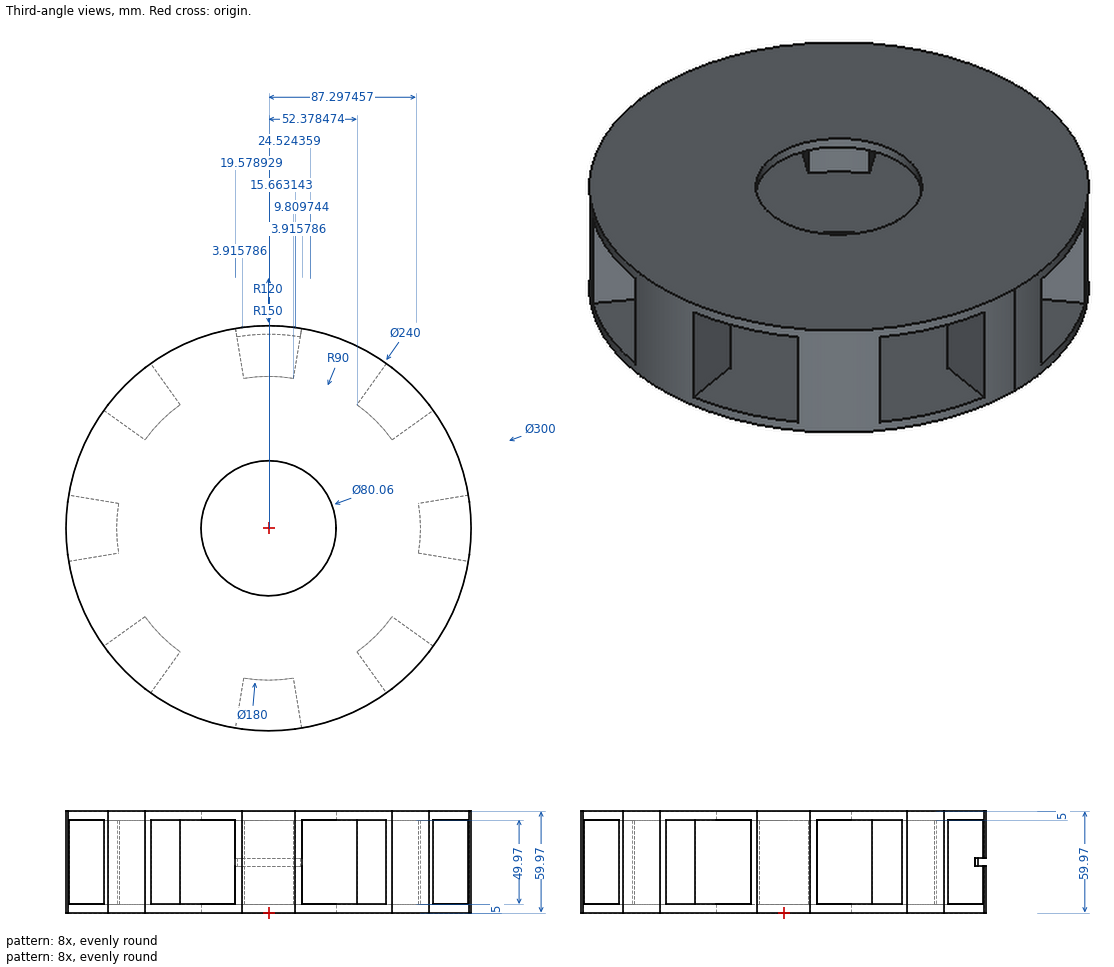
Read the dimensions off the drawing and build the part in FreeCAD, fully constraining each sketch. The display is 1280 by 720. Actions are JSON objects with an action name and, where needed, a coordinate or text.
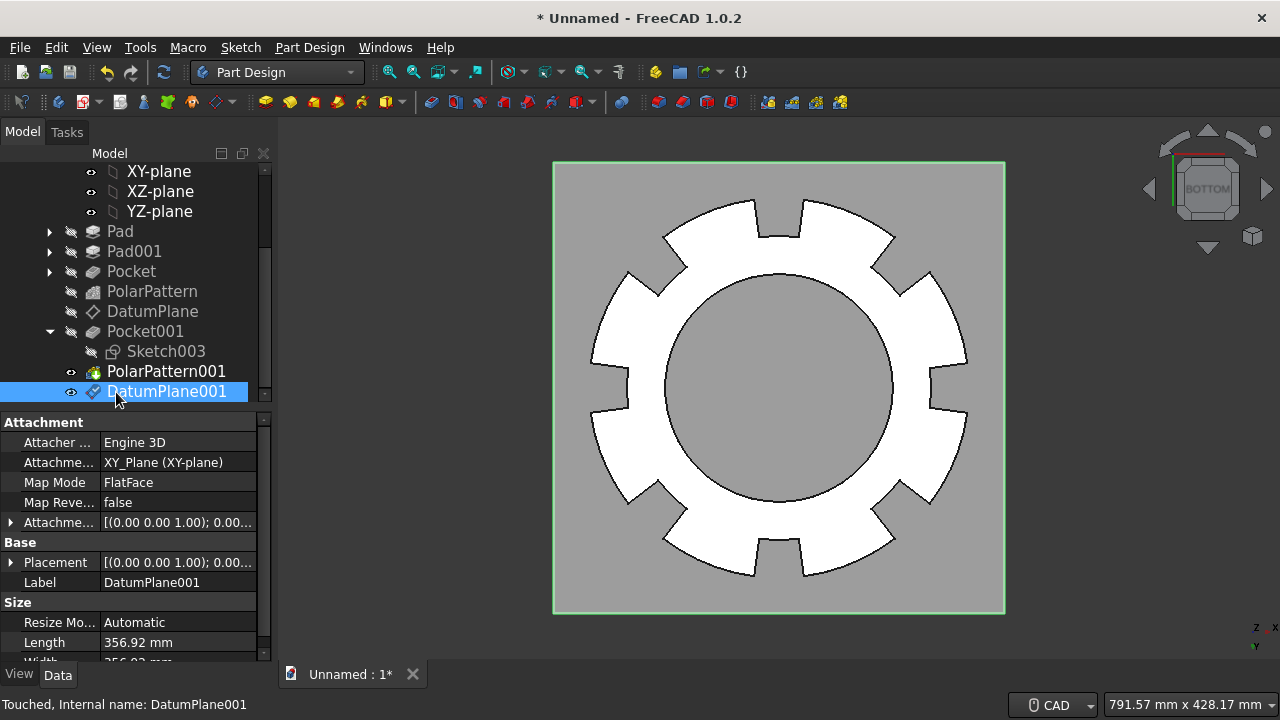
{"action": "left_click", "coordinate": [84, 102]}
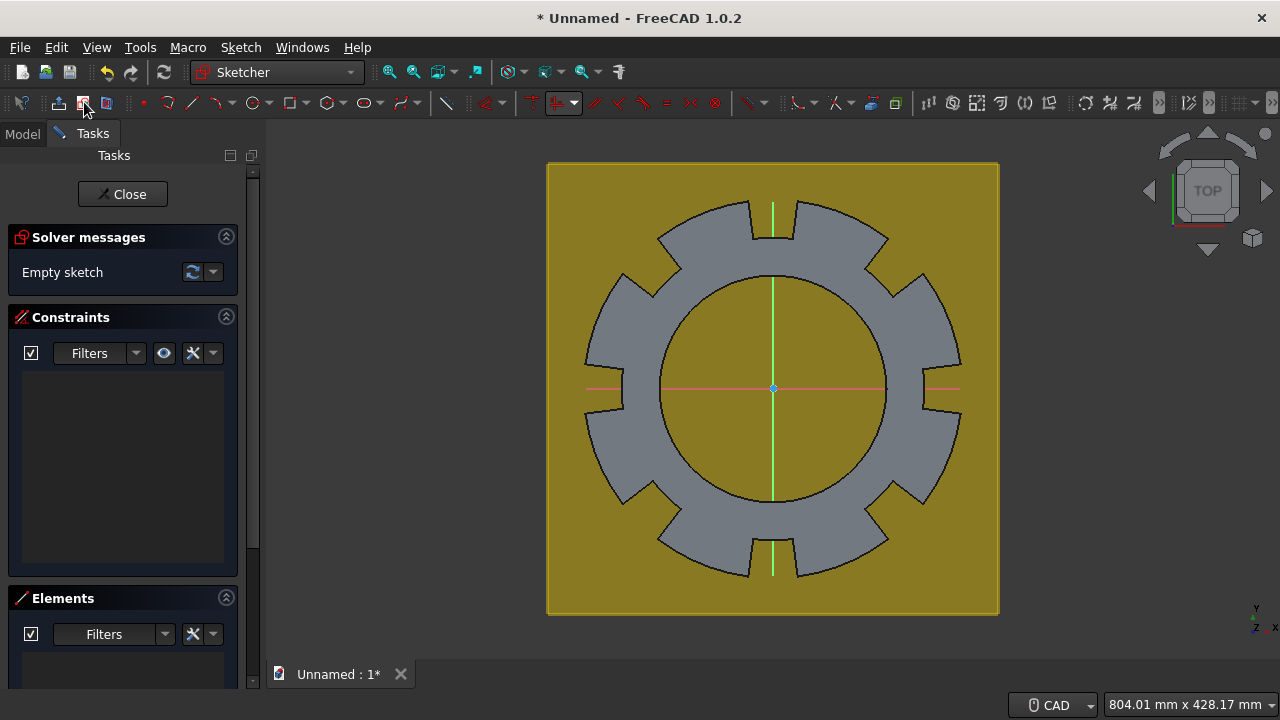
{"action": "left_click", "coordinate": [108, 104]}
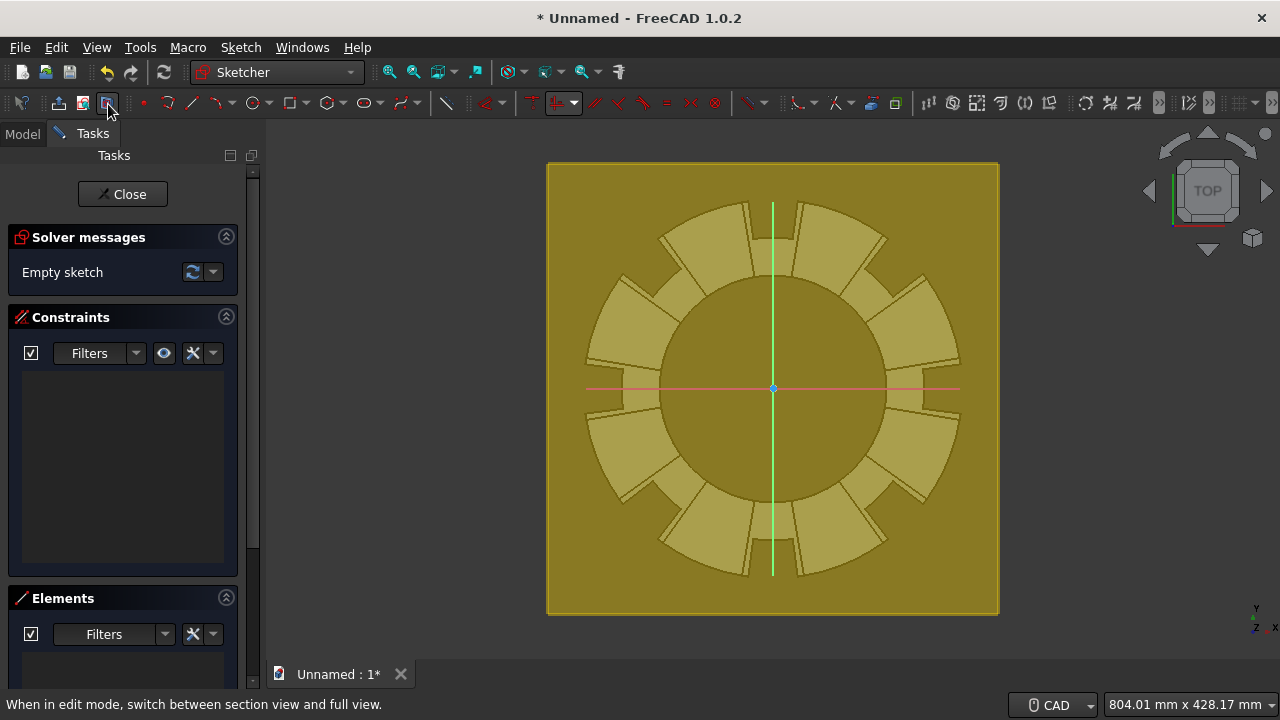
{"action": "scroll", "coordinate": [912, 389], "scroll_direction": "up", "scroll_amount": 2}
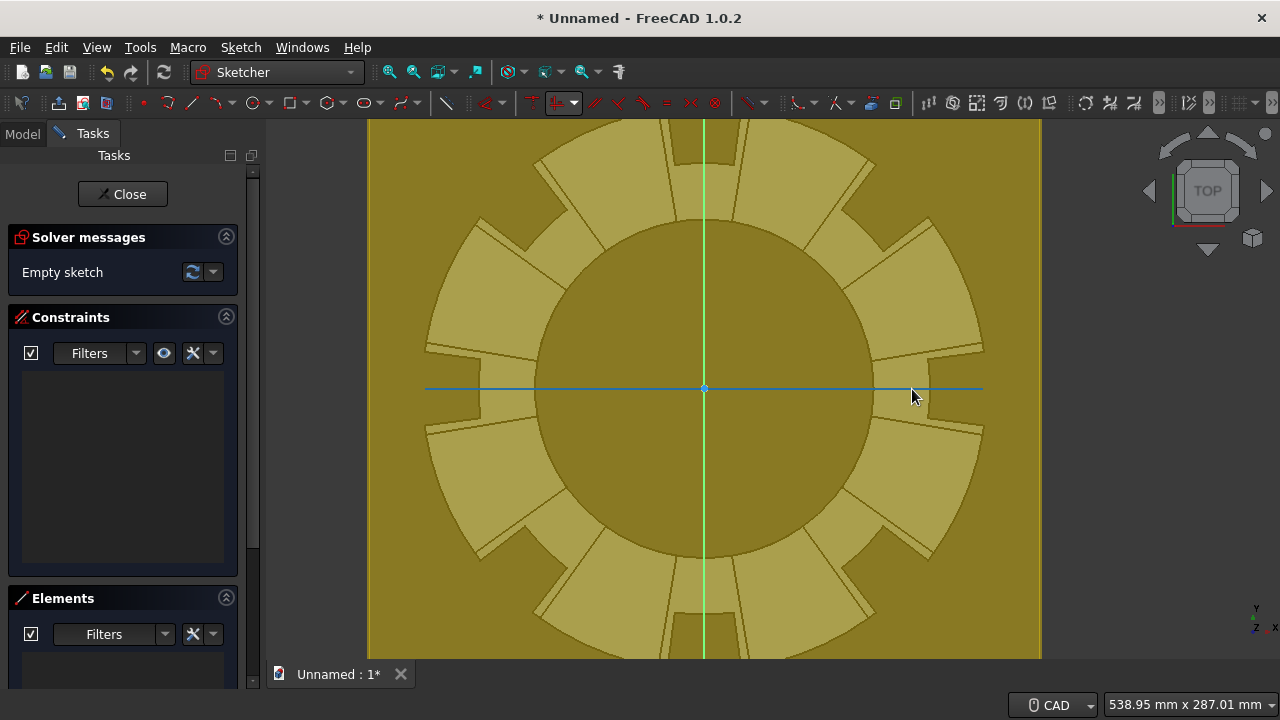
{"action": "left_click", "coordinate": [254, 104]}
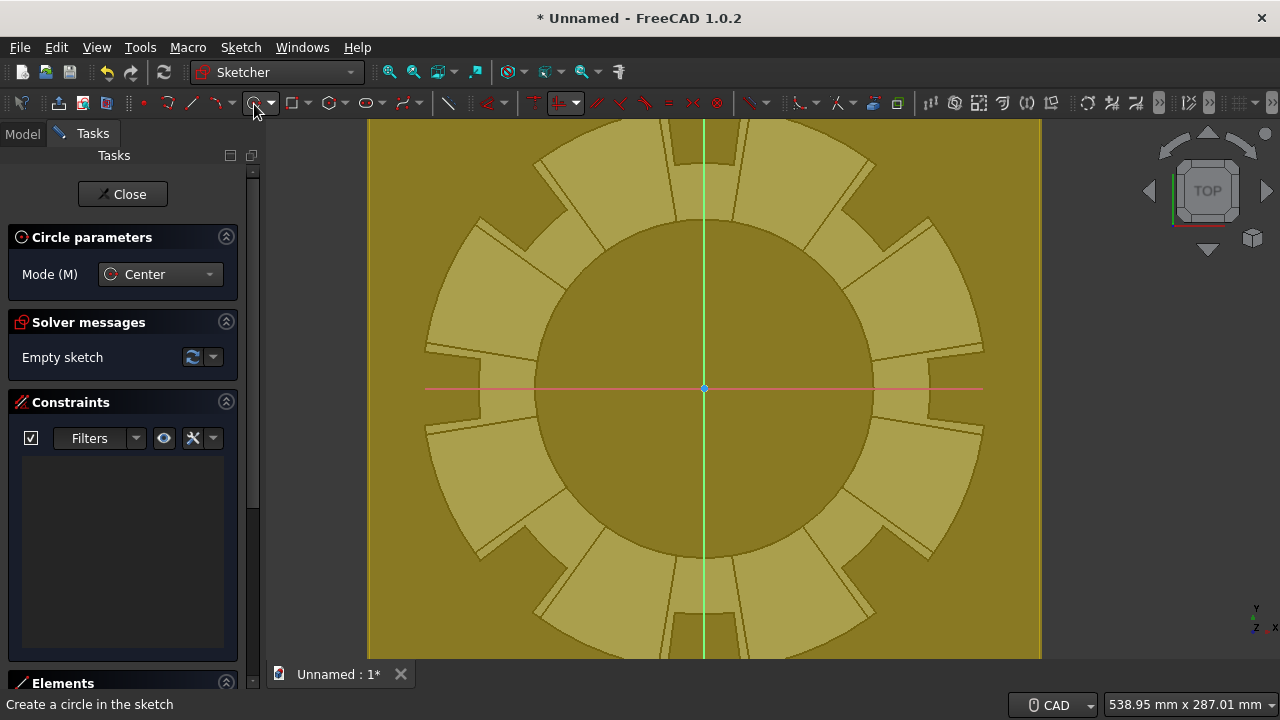
{"action": "left_click", "coordinate": [704, 389]}
{"action": "left_click", "coordinate": [824, 269]}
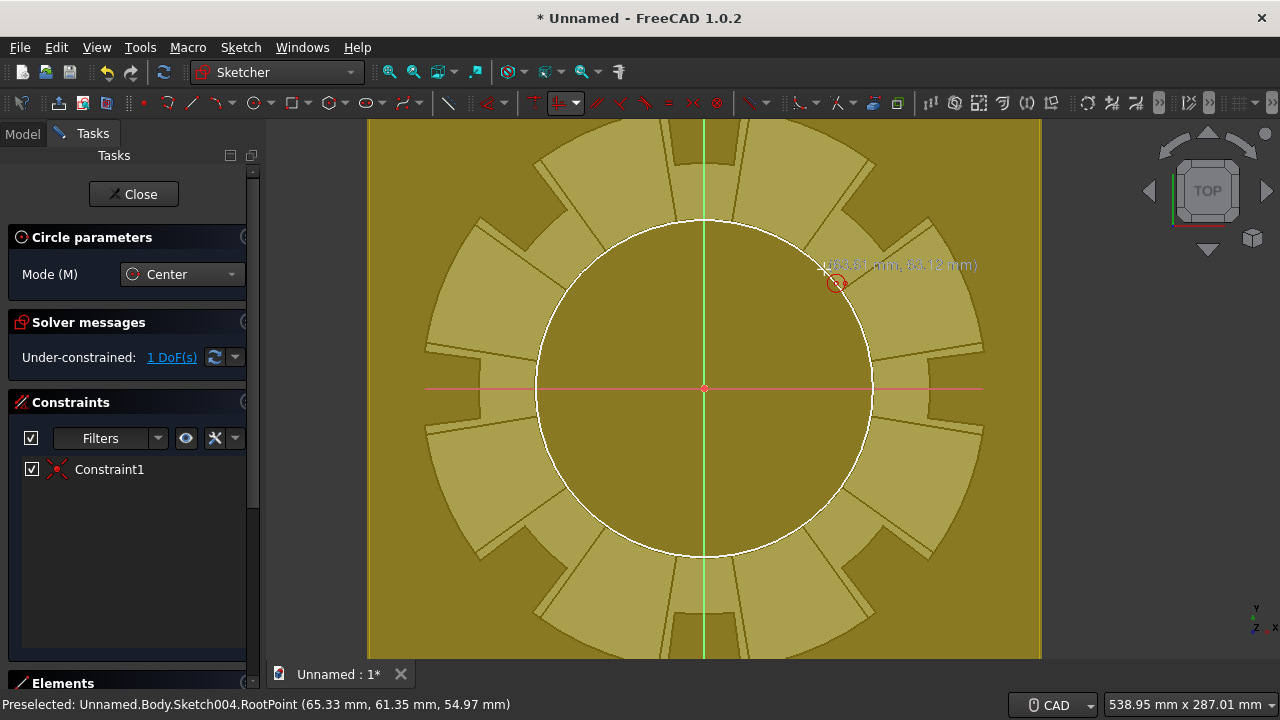
{"action": "left_click", "coordinate": [704, 389]}
{"action": "left_click", "coordinate": [758, 335]}
{"action": "key", "text": "Escape"}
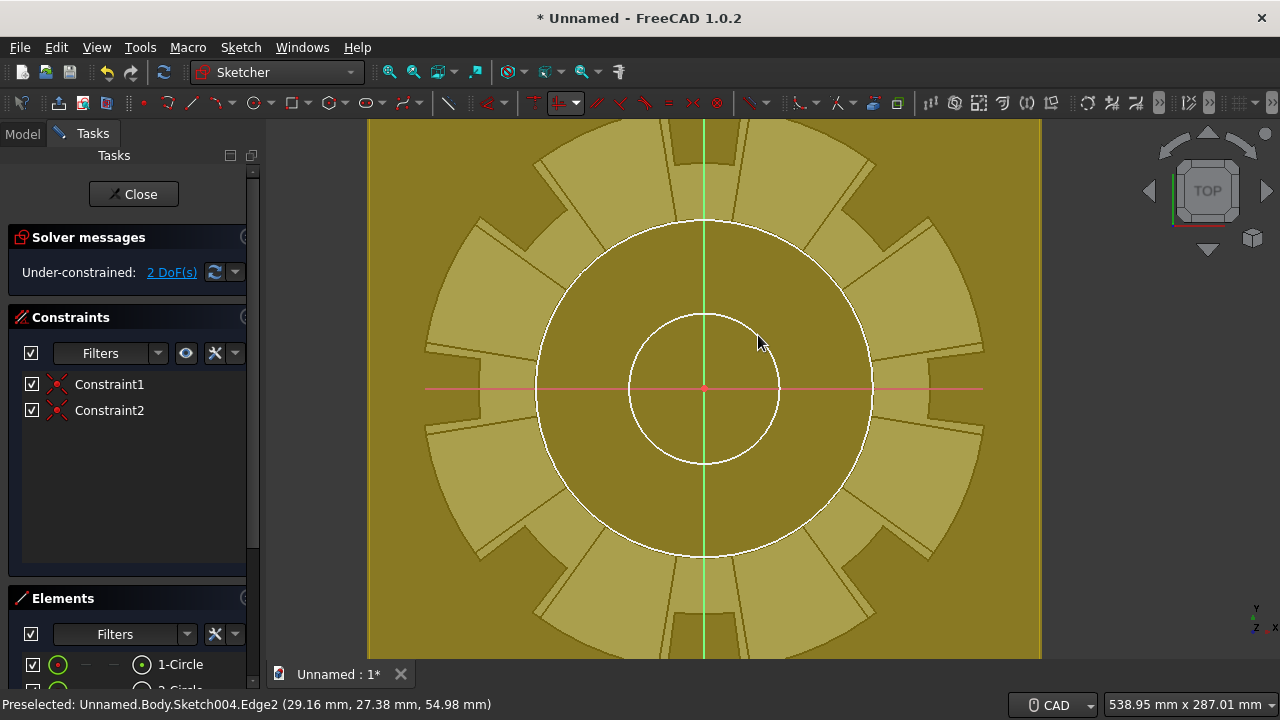
{"action": "key", "text": "d"}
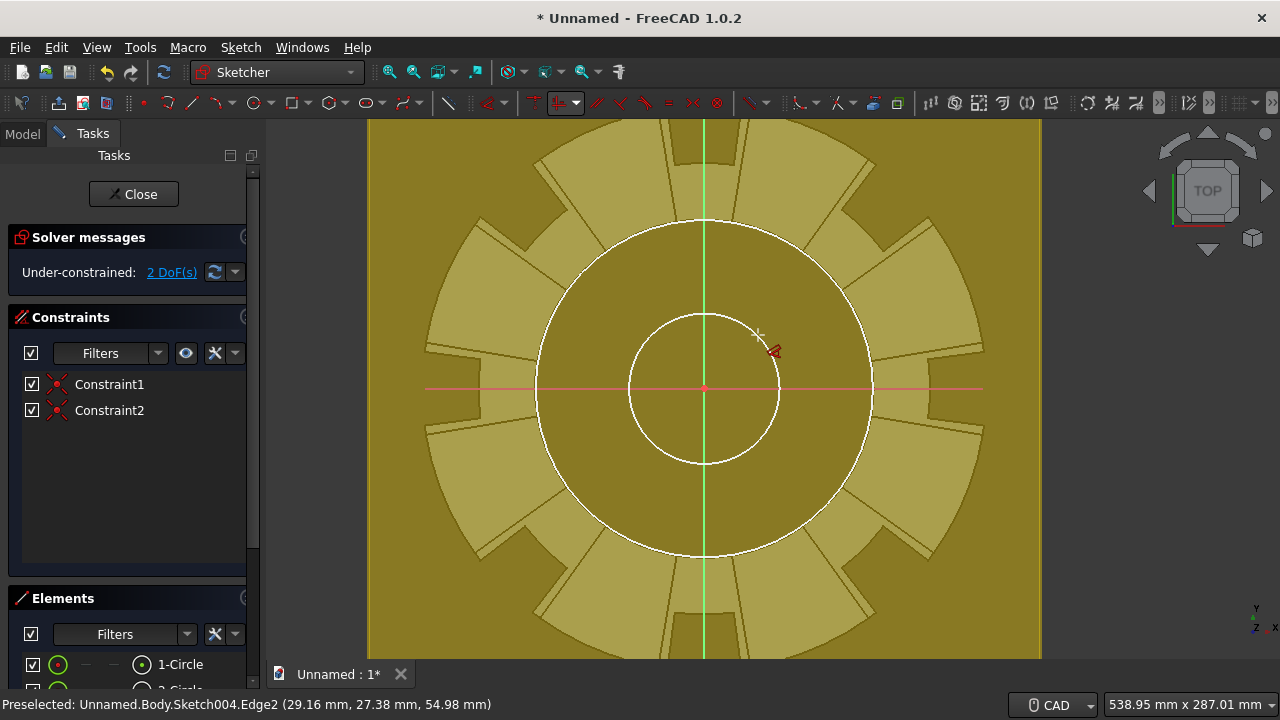
{"action": "left_click", "coordinate": [823, 269]}
{"action": "left_click", "coordinate": [846, 246]}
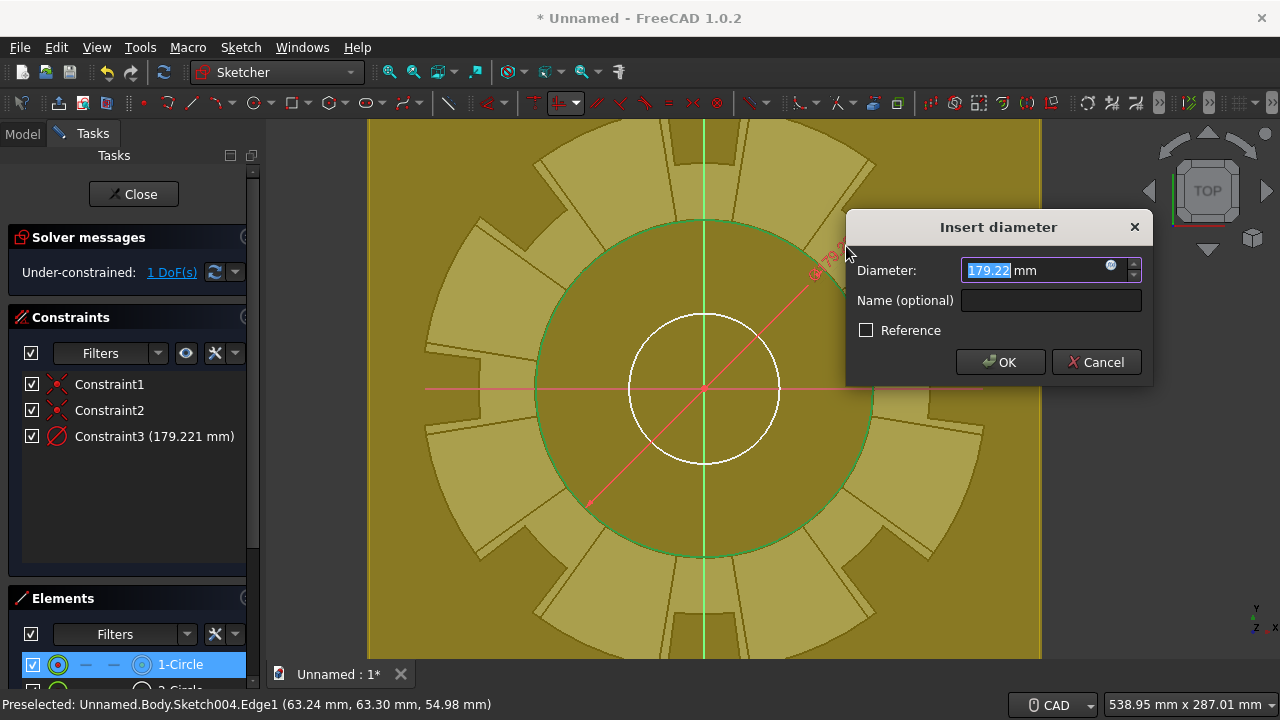
{"action": "type", "text": "180"}
{"action": "key", "text": "Return"}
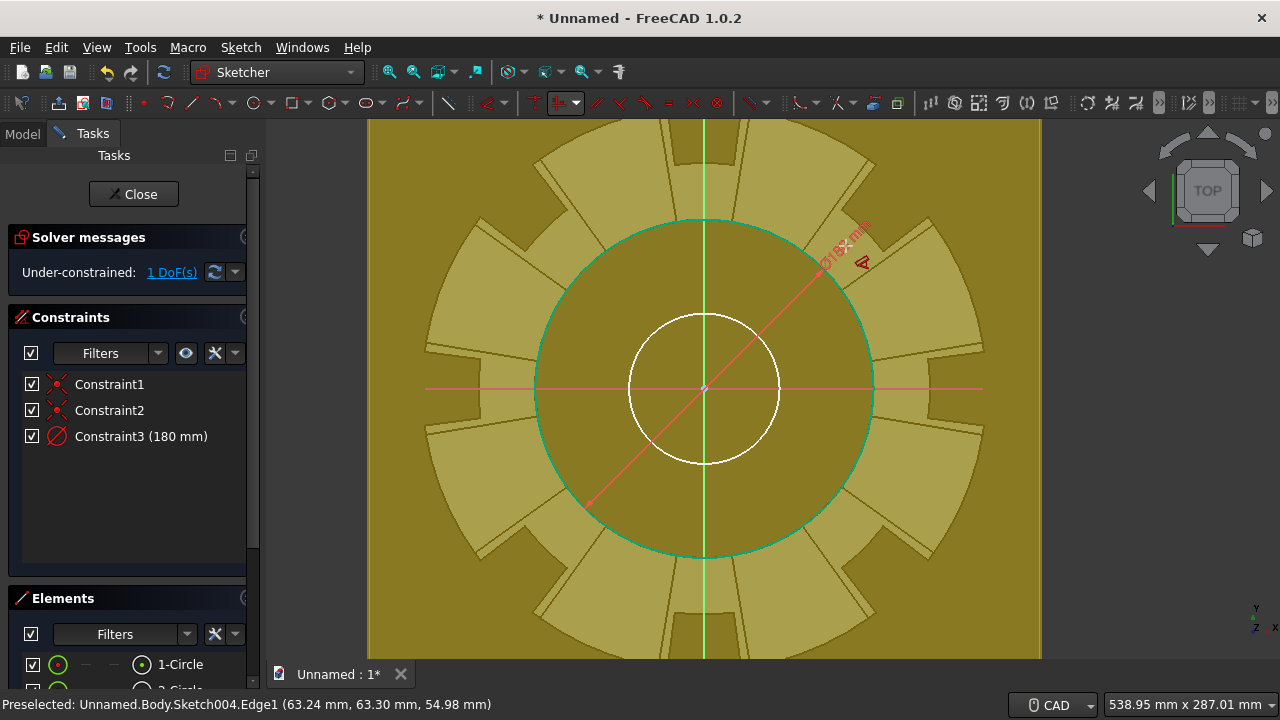
{"action": "left_click", "coordinate": [757, 335]}
{"action": "left_click", "coordinate": [779, 312]}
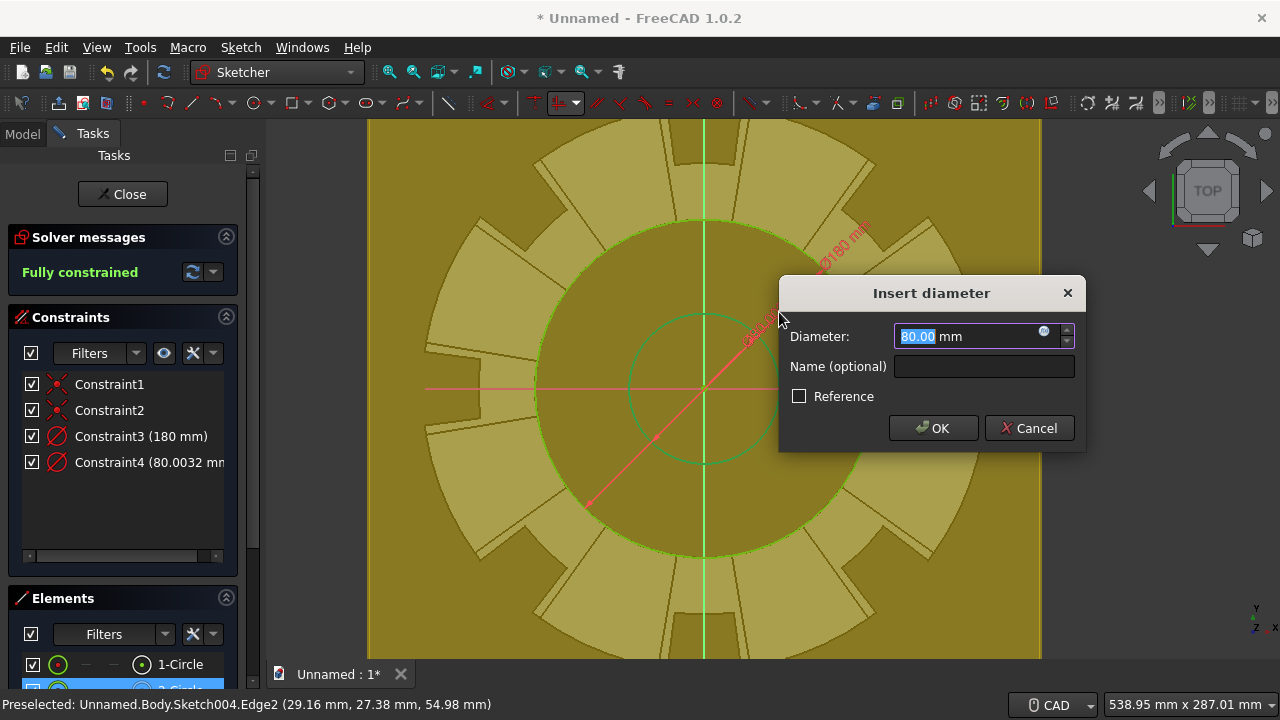
{"action": "type", "text": "80.06"}
{"action": "key", "text": "Return"}
{"action": "key", "text": "Escape"}